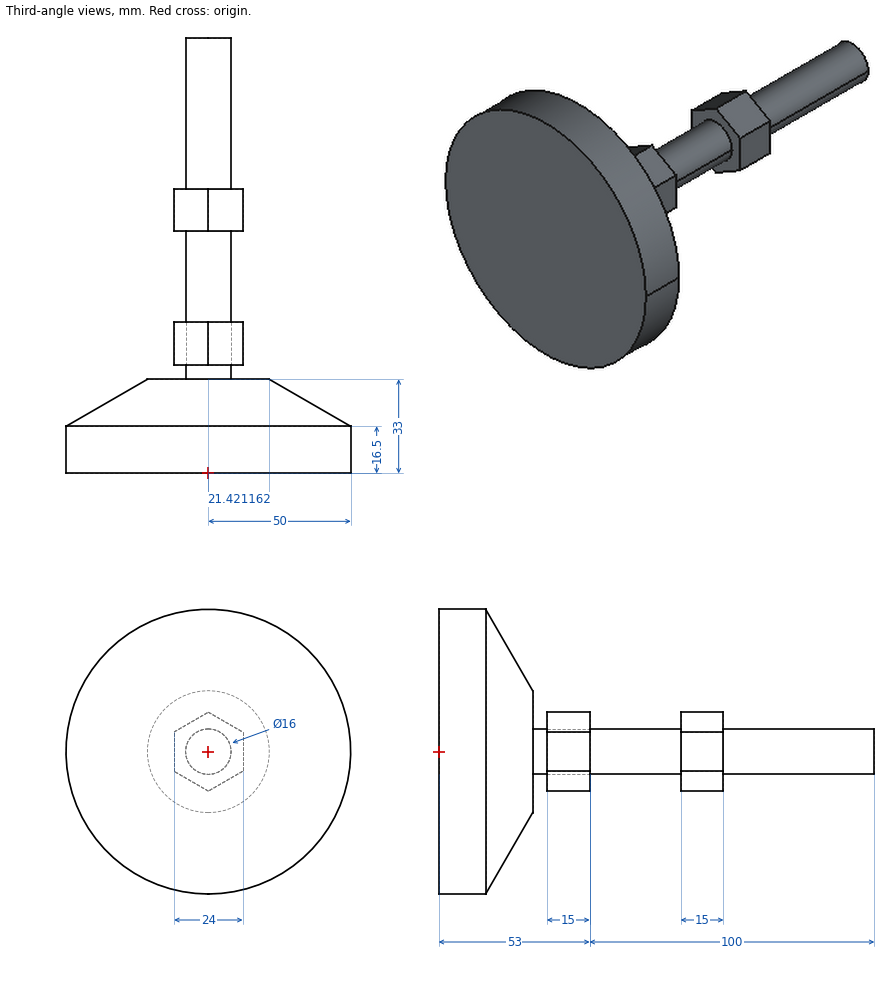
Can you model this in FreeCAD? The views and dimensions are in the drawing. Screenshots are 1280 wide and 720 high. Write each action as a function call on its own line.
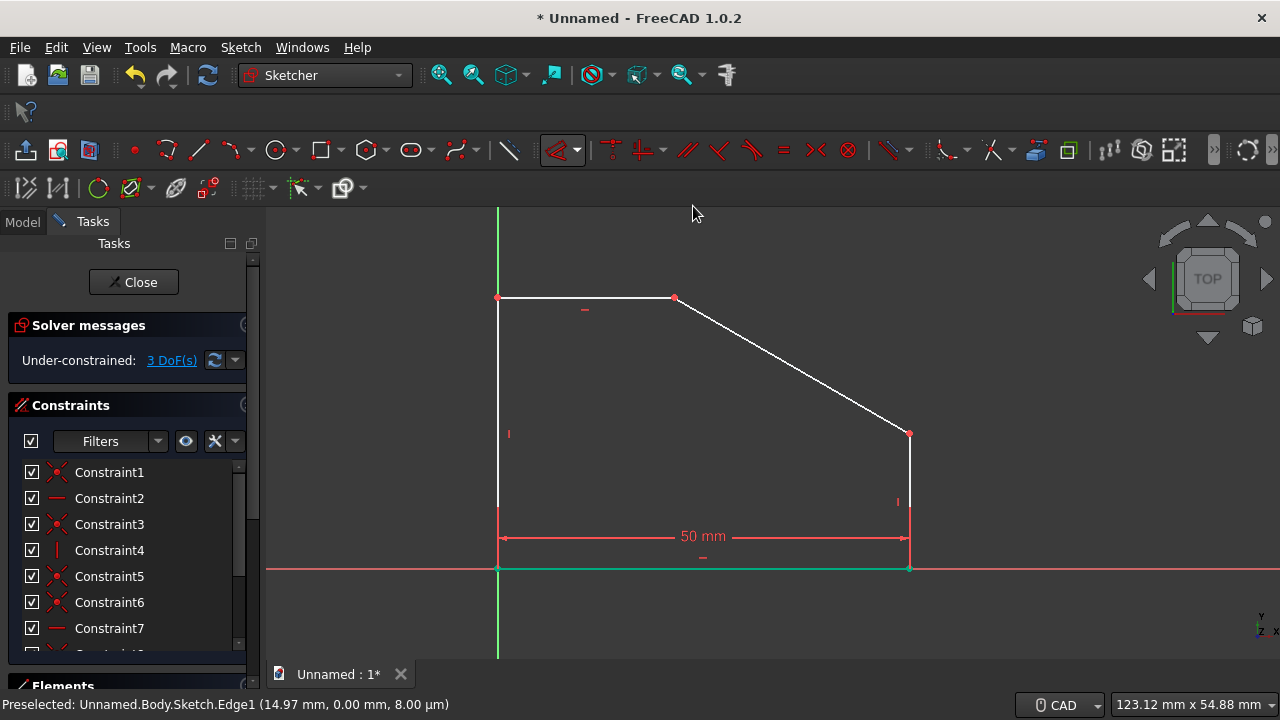
click(498, 379)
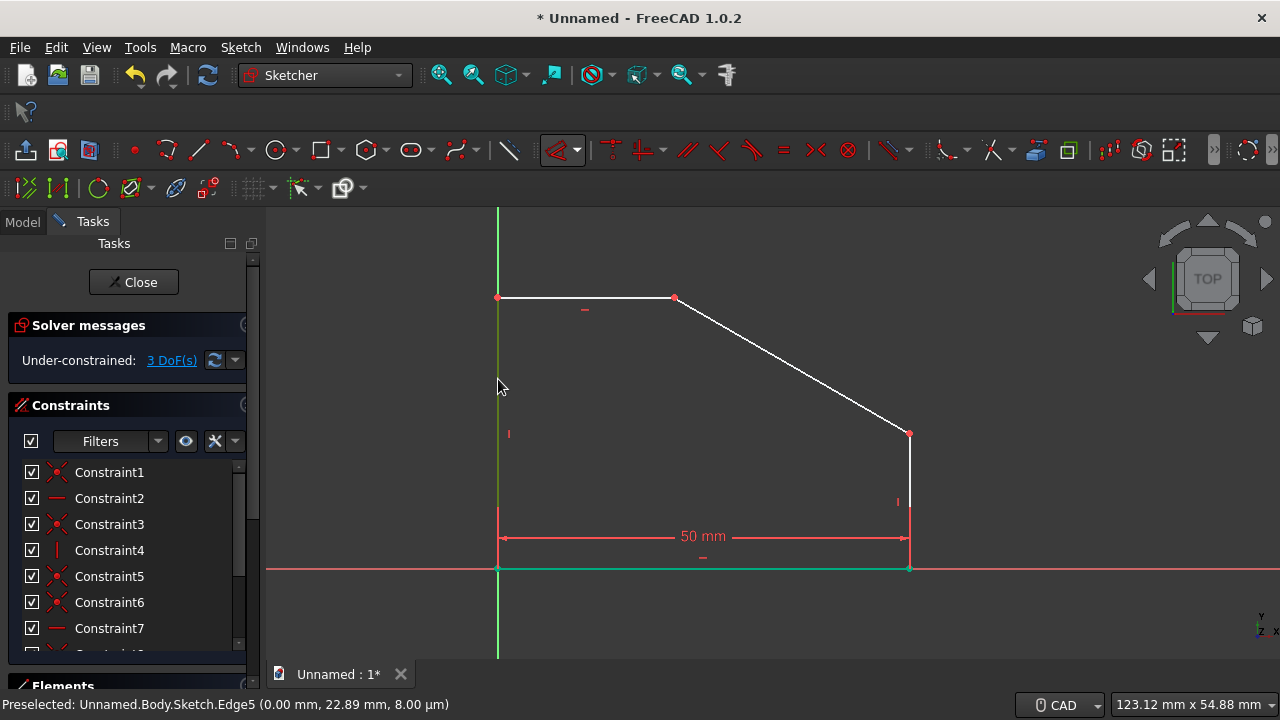
key(i)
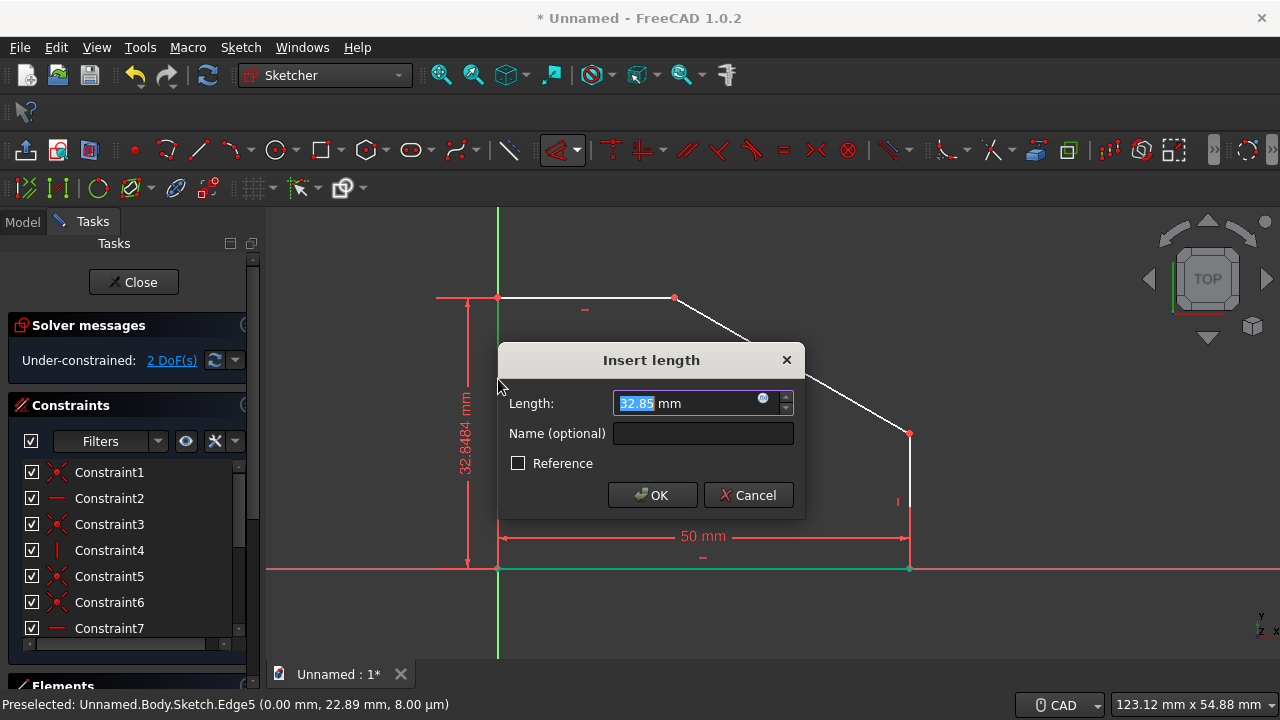
text(33)
key(Return)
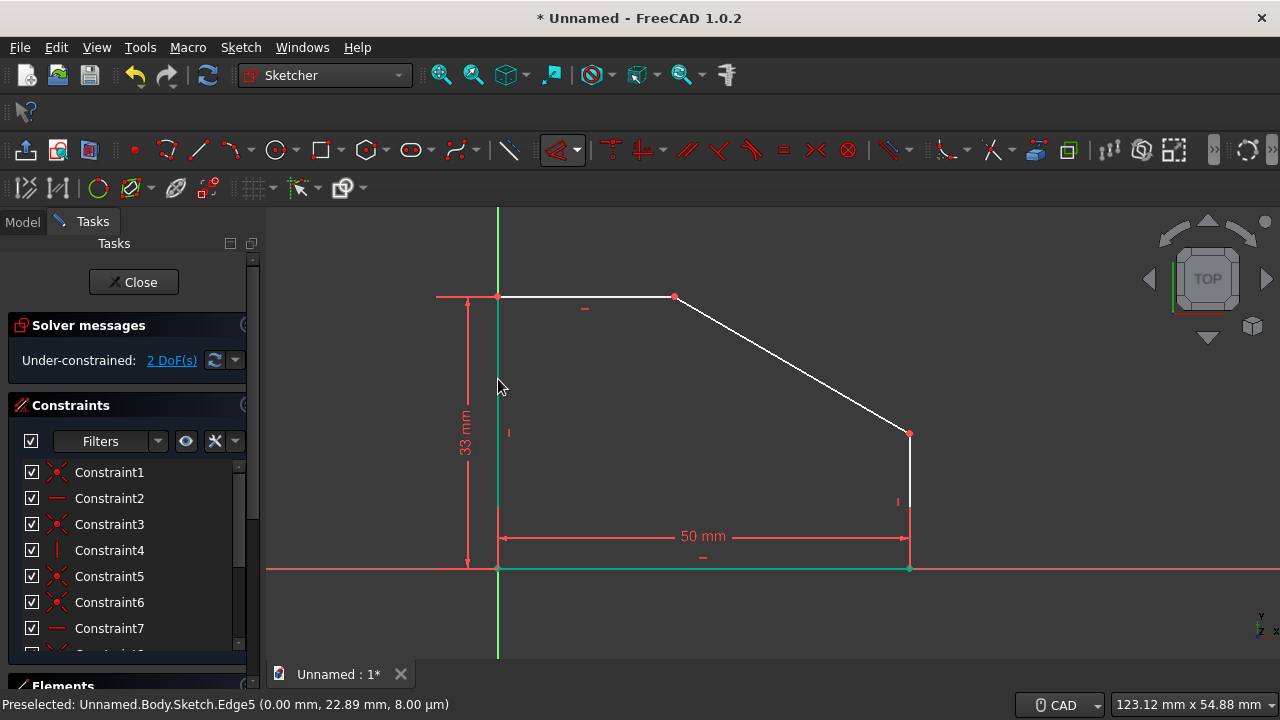
click(910, 528)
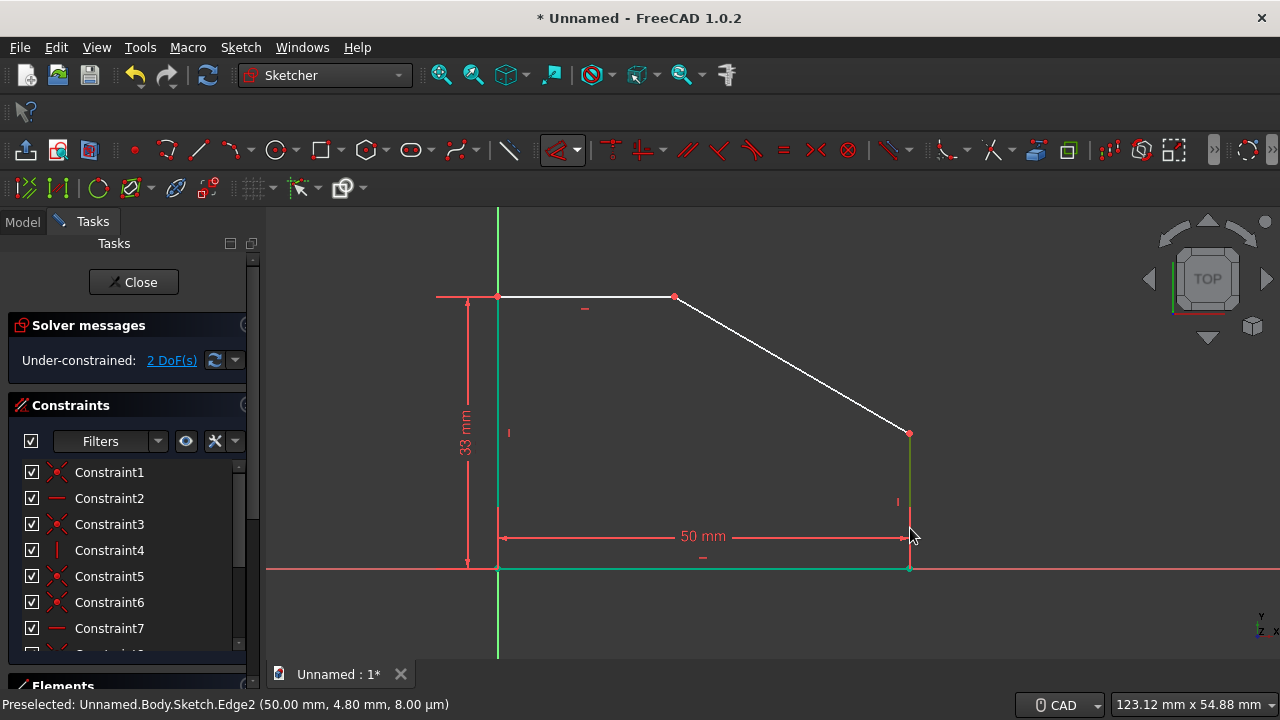
key(i)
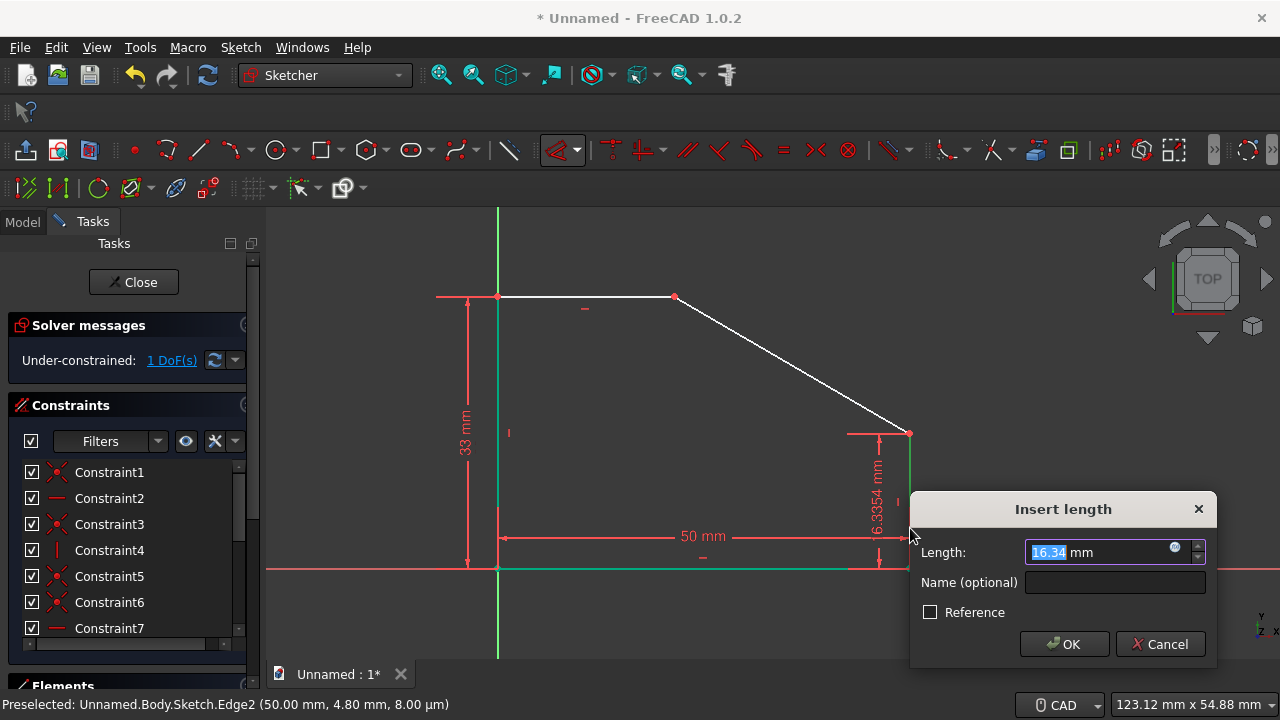
text(16.5)
key(Return)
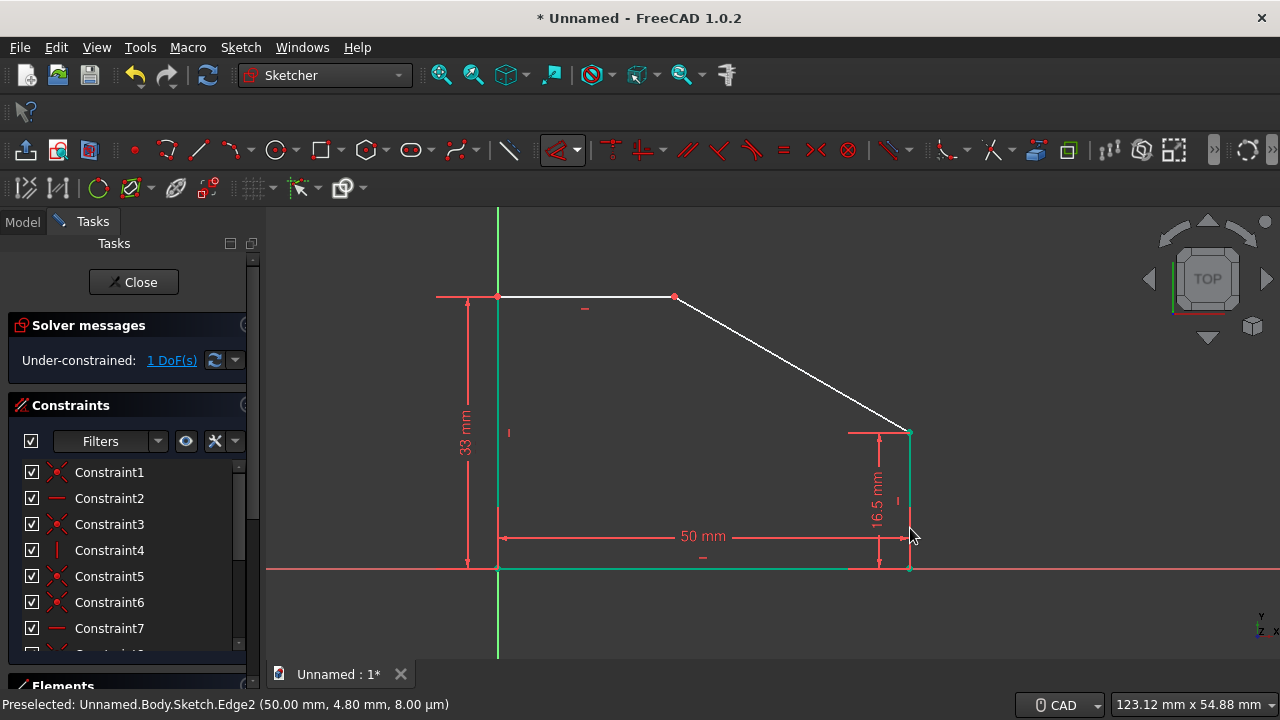
click(621, 297)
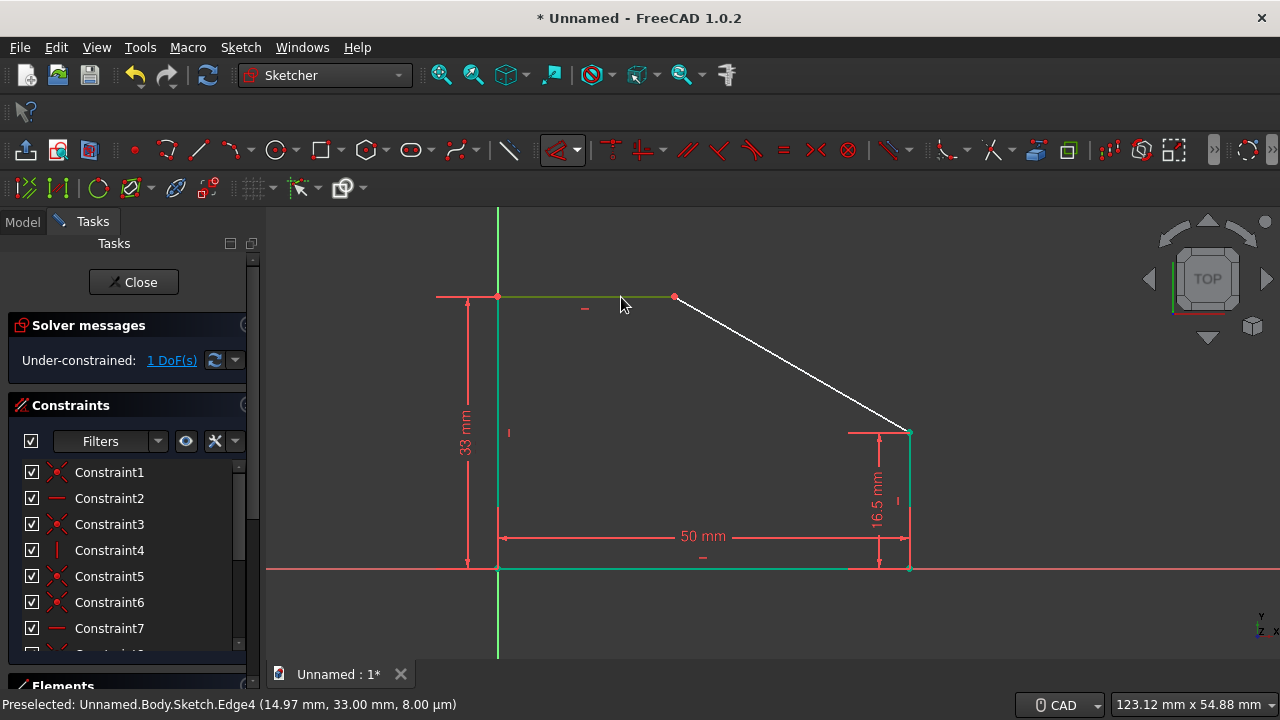
key(l)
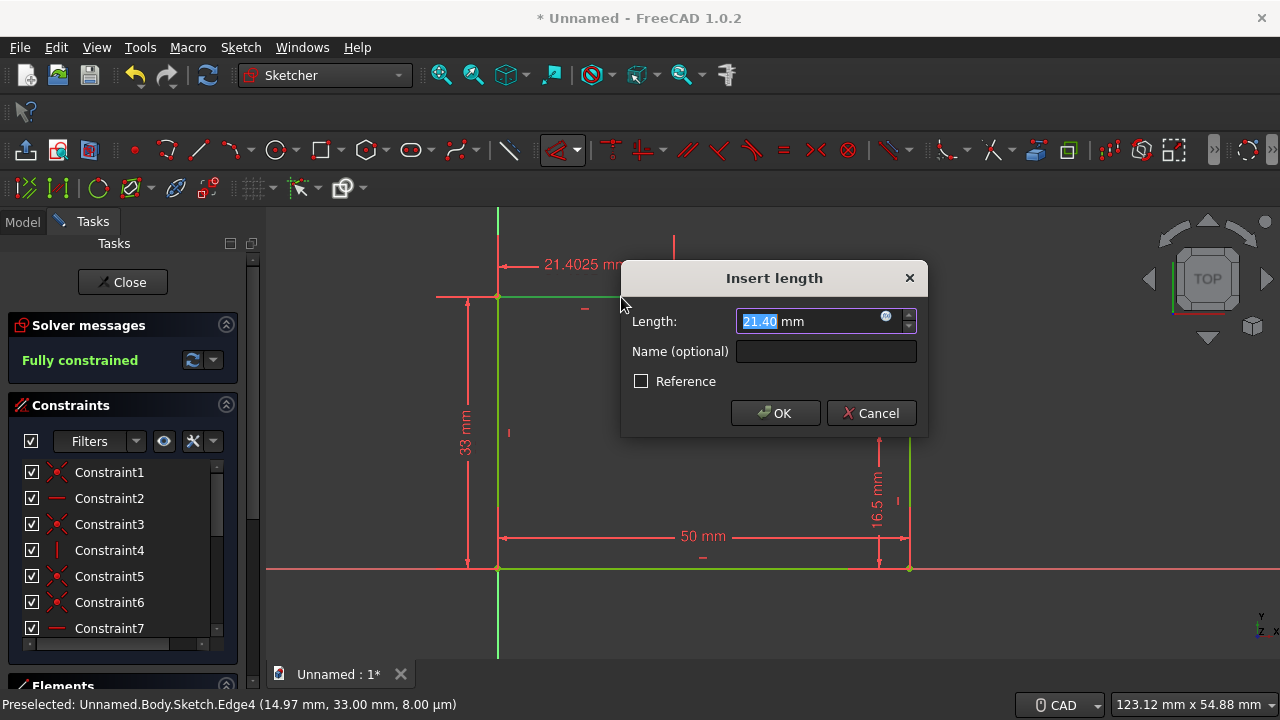
text(21.421162)
key(Return)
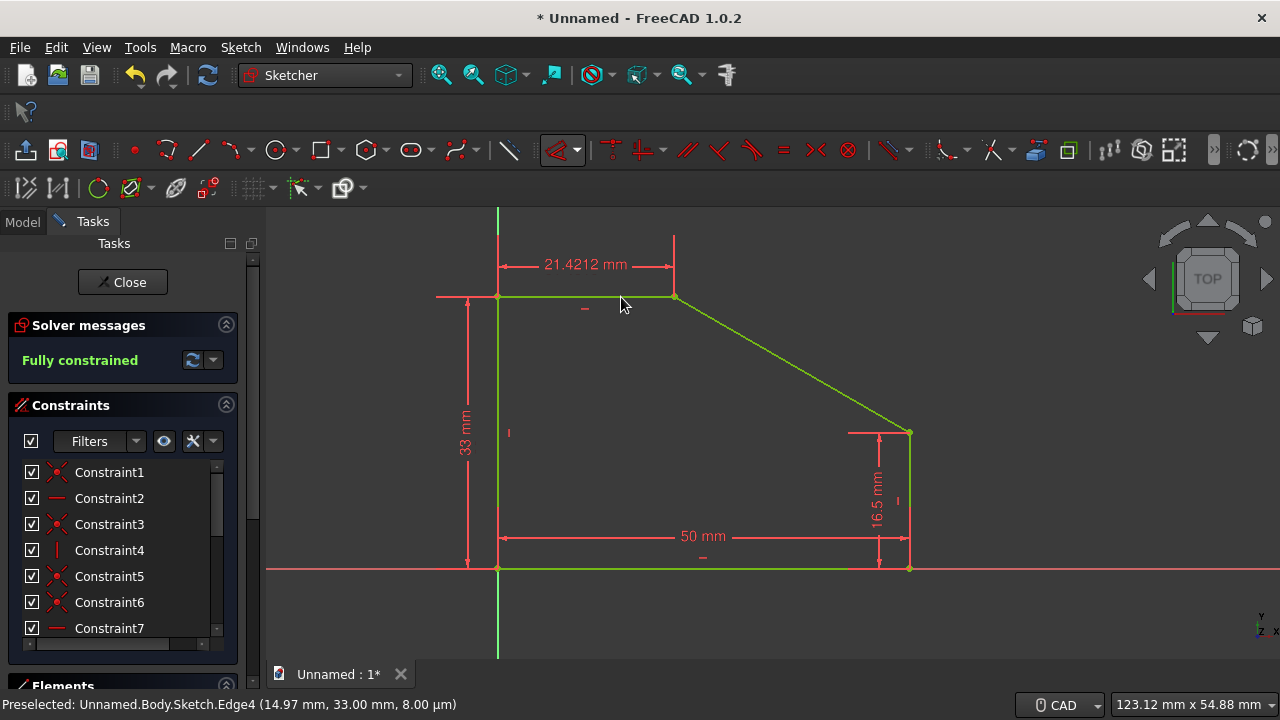
click(123, 282)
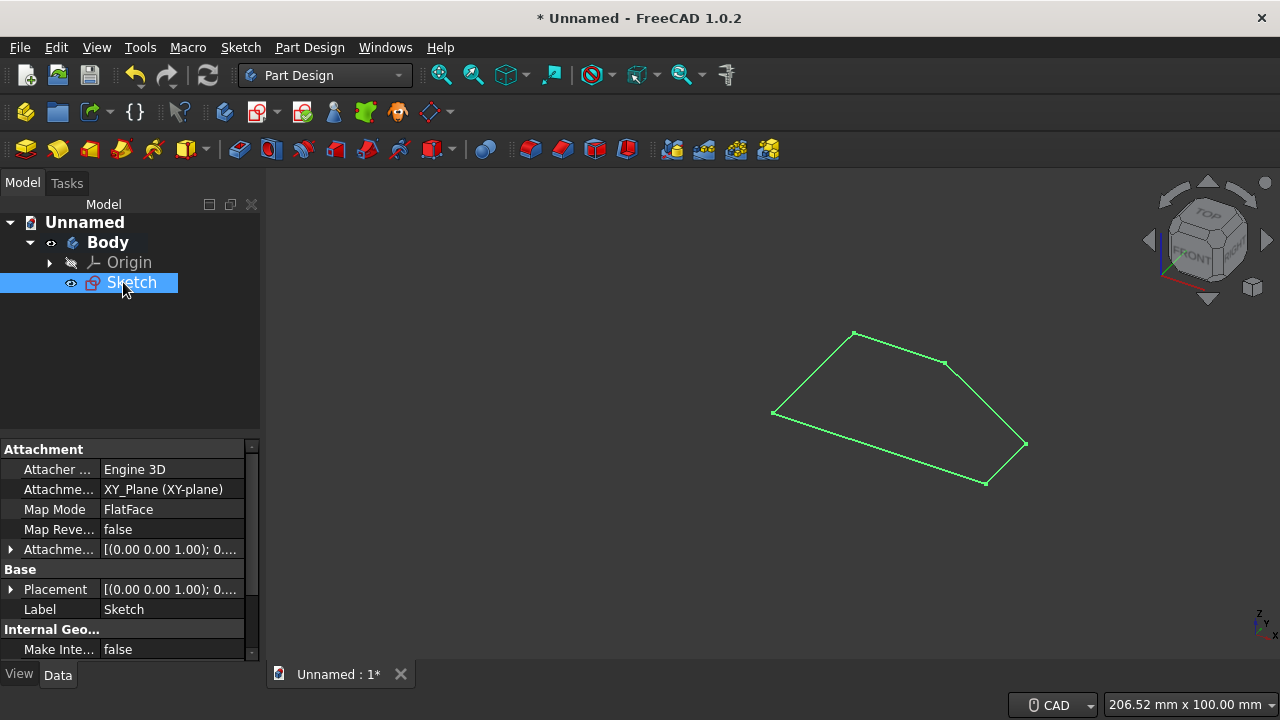
click(58, 150)